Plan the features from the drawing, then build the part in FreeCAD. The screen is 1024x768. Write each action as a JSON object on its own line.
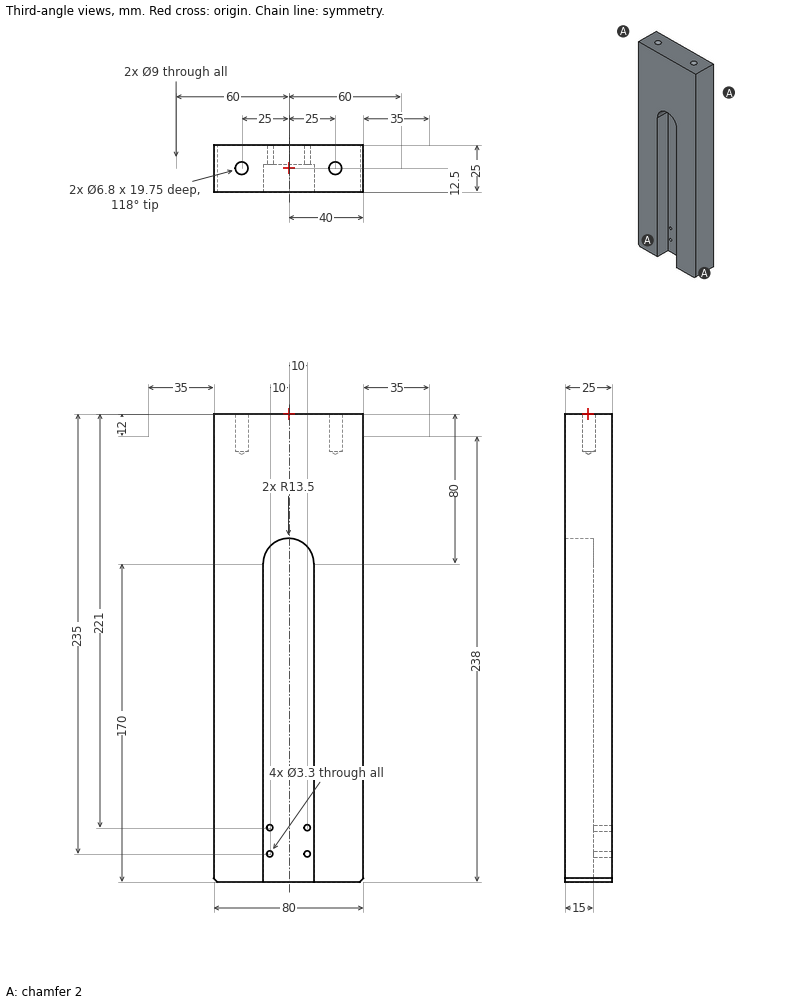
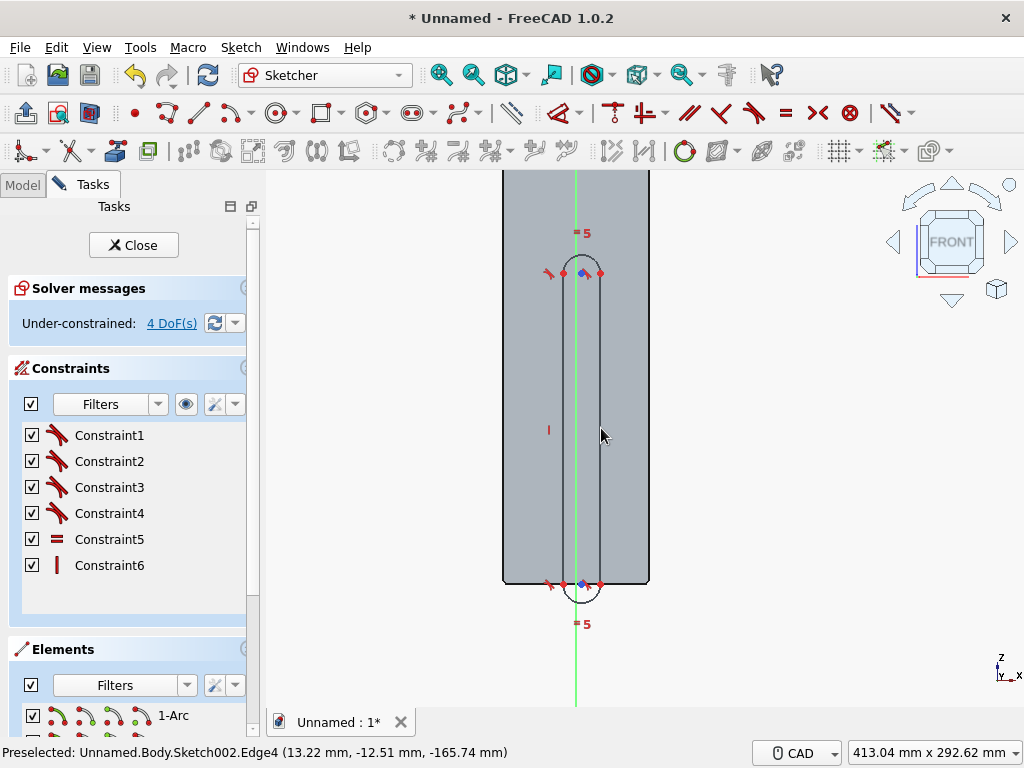
{"action": "left_click", "coordinate": [582, 585]}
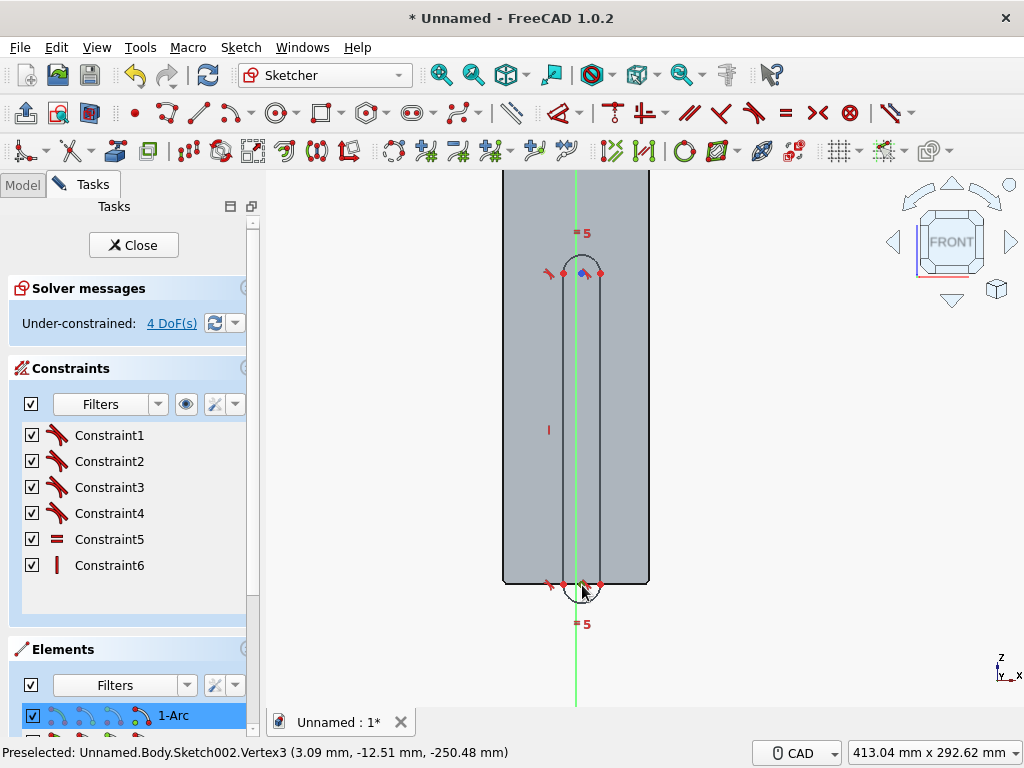
{"action": "left_click", "coordinate": [576, 645]}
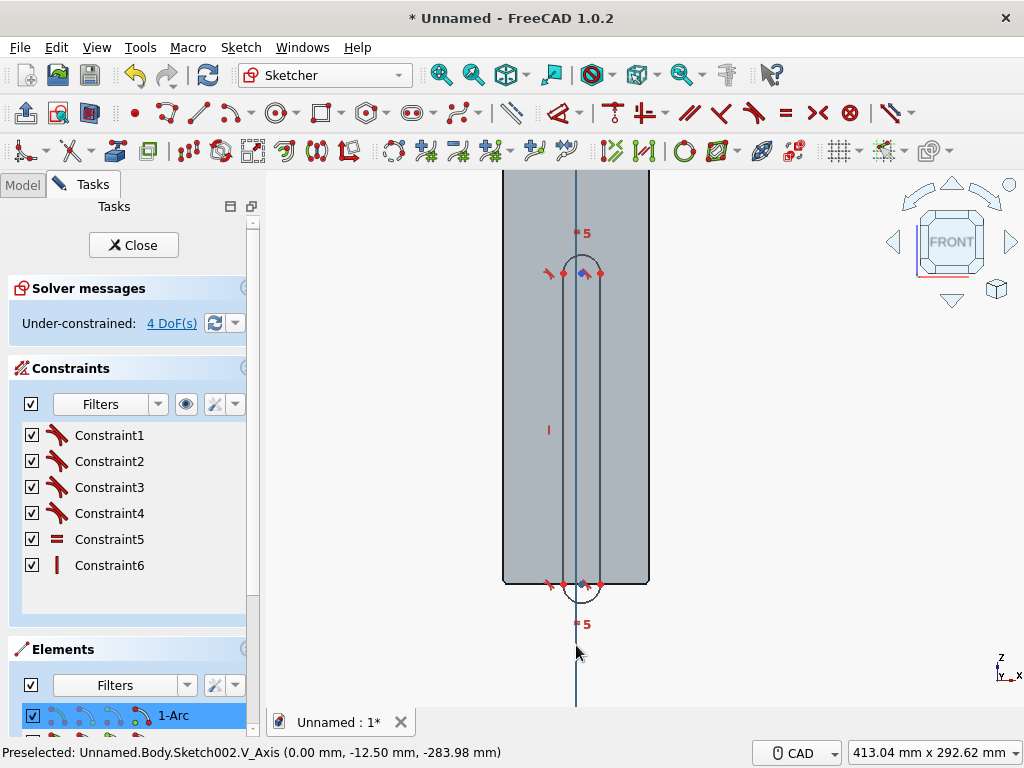
{"action": "left_click", "coordinate": [614, 114]}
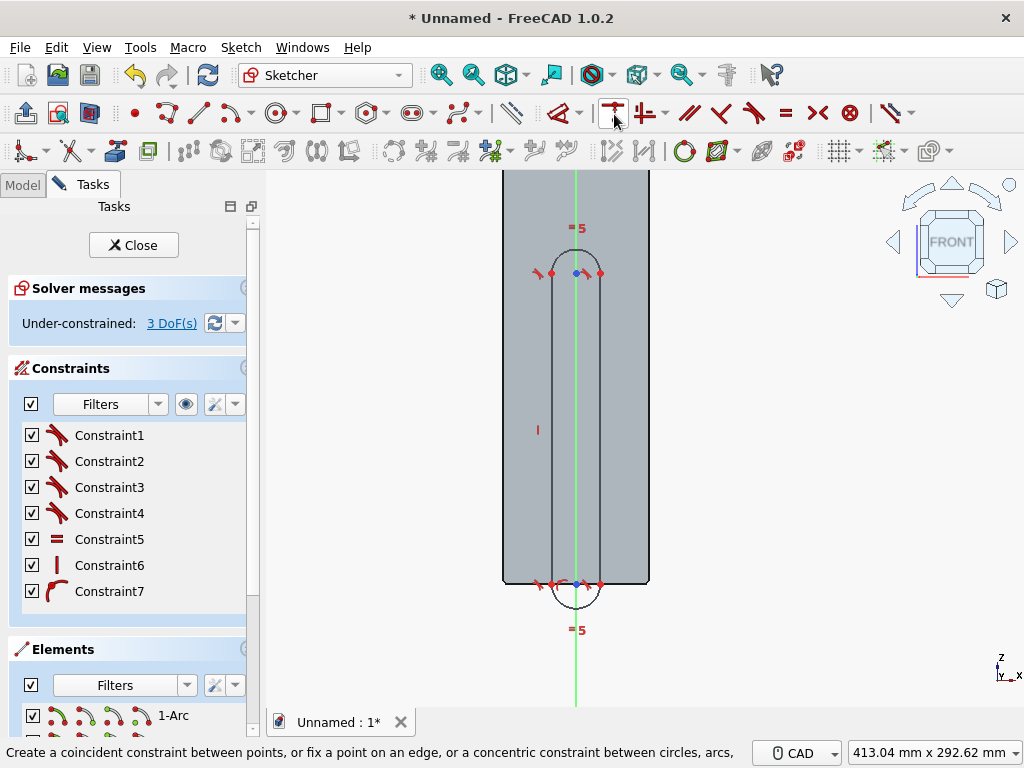
{"action": "left_click", "coordinate": [558, 114]}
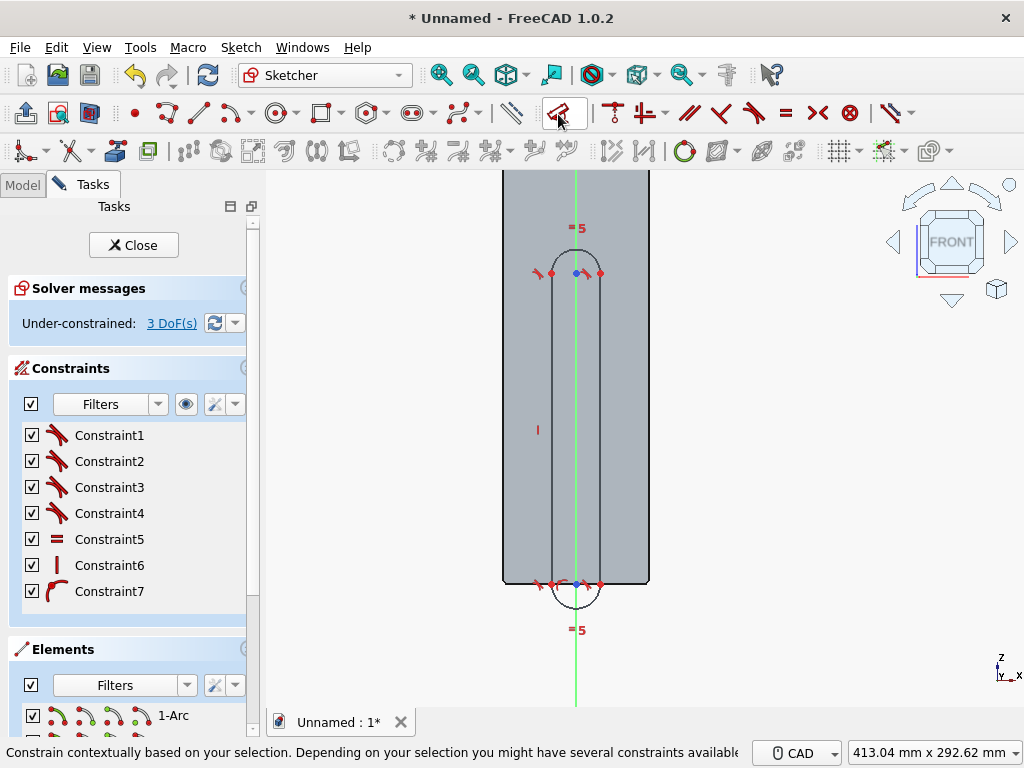
{"action": "scroll", "coordinate": [562, 604], "scroll_direction": "up", "scroll_amount": 3}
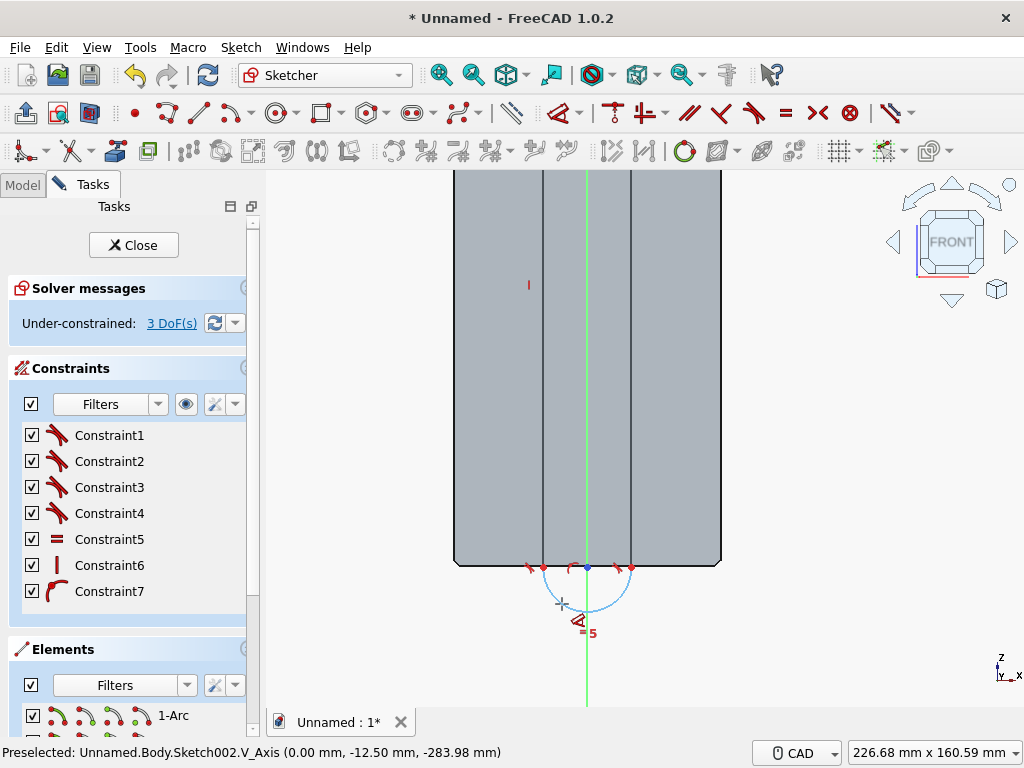
{"action": "left_click", "coordinate": [561, 603]}
{"action": "left_click", "coordinate": [542, 629]}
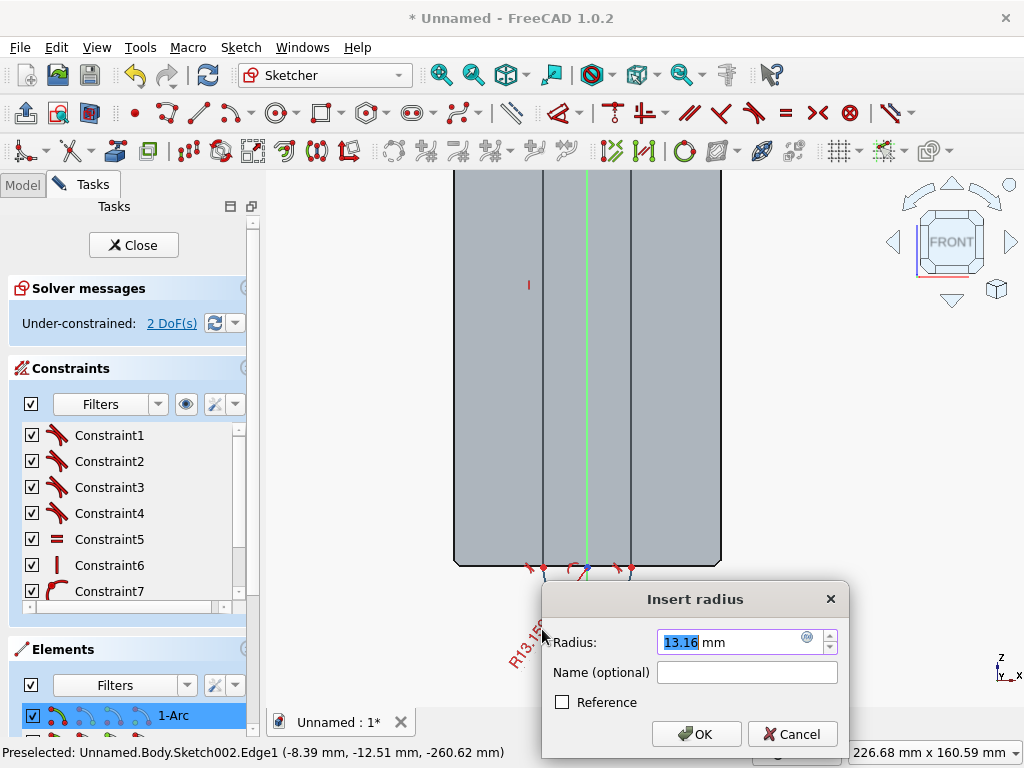
{"action": "type", "text": "13.5"}
{"action": "key", "text": "Return"}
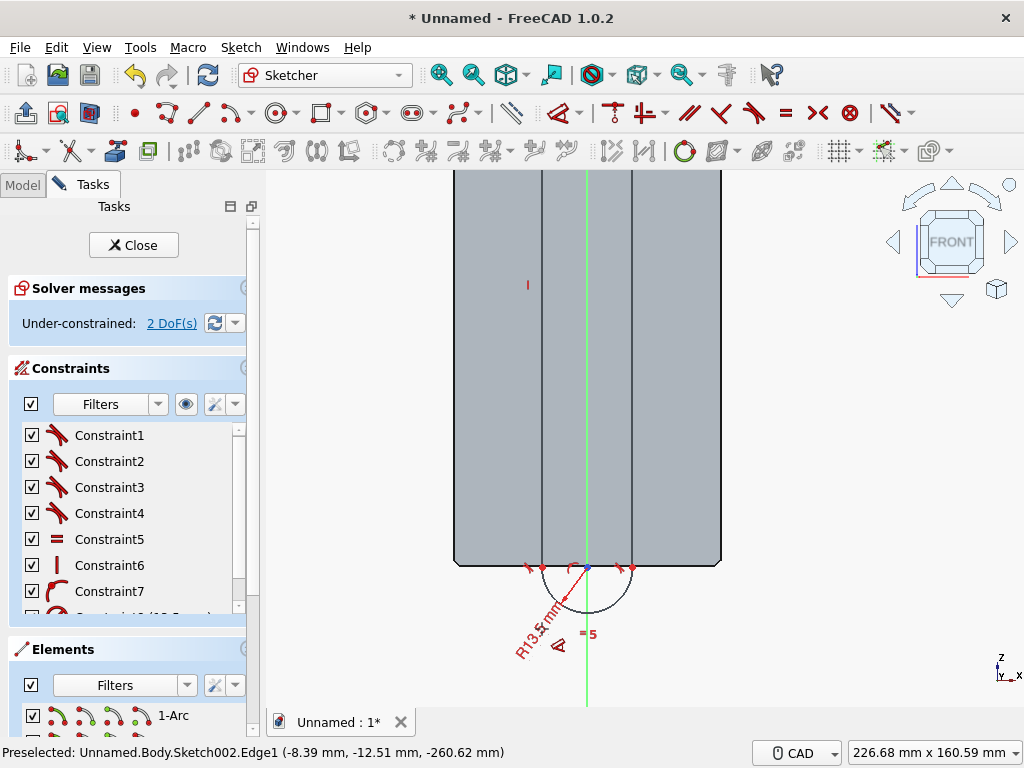
{"action": "left_click", "coordinate": [542, 398]}
{"action": "left_click", "coordinate": [508, 383]}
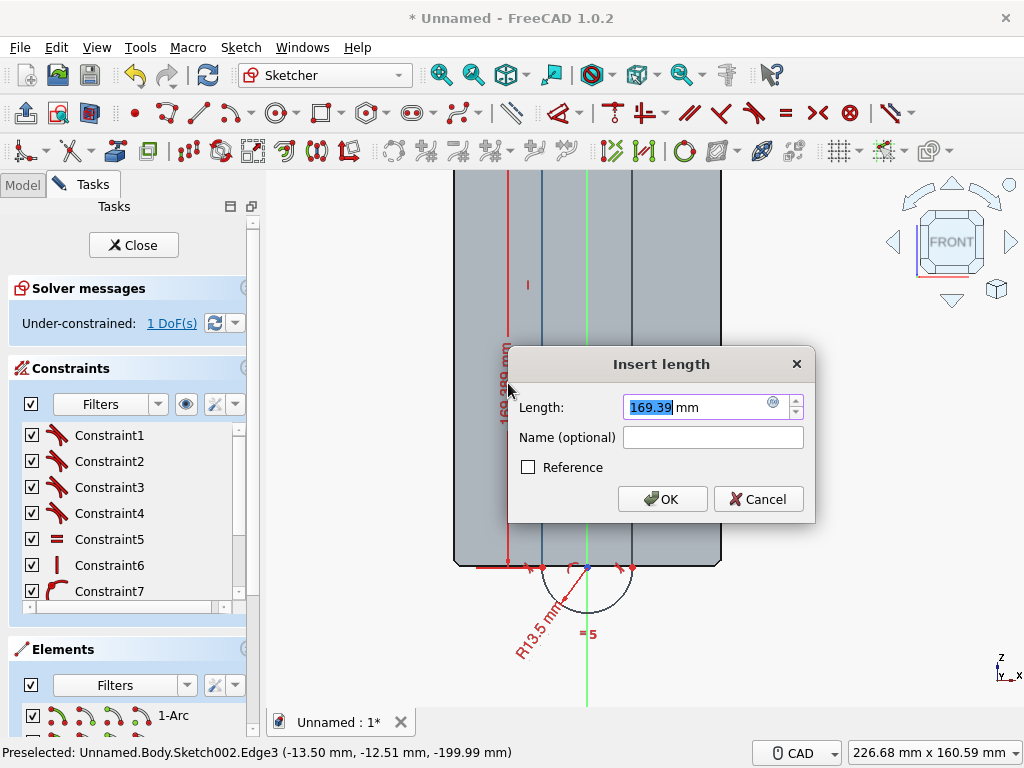
{"action": "type", "text": "170"}
{"action": "key", "text": "Return"}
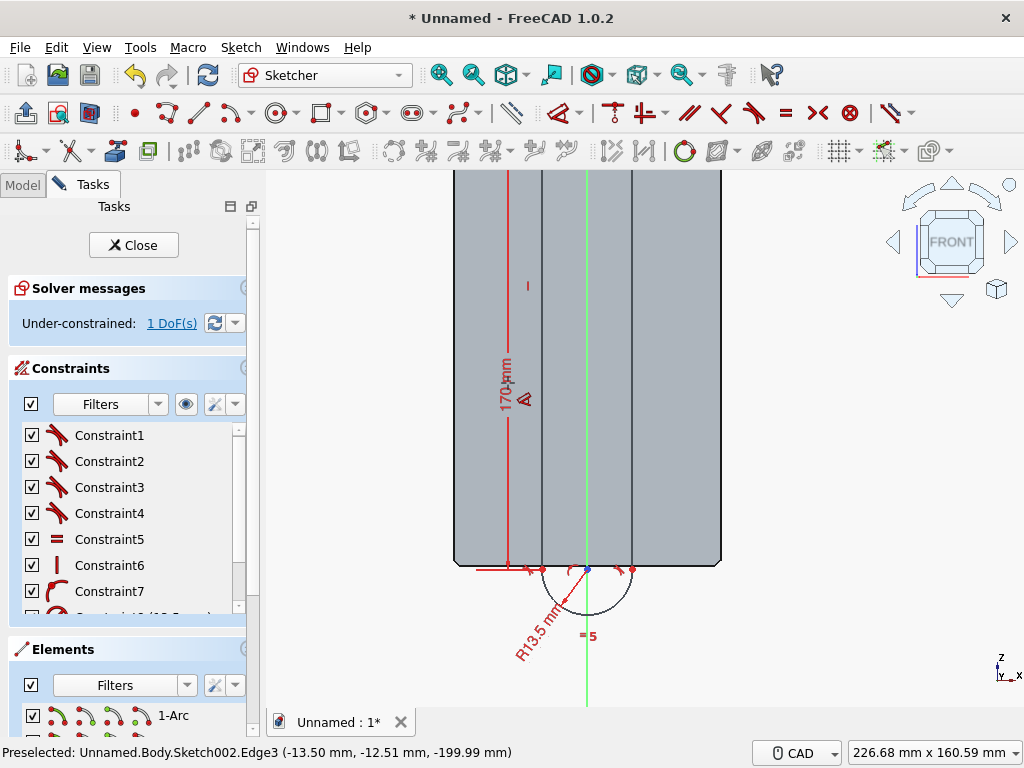
{"action": "scroll", "coordinate": [570, 594], "scroll_direction": "down", "scroll_amount": 5}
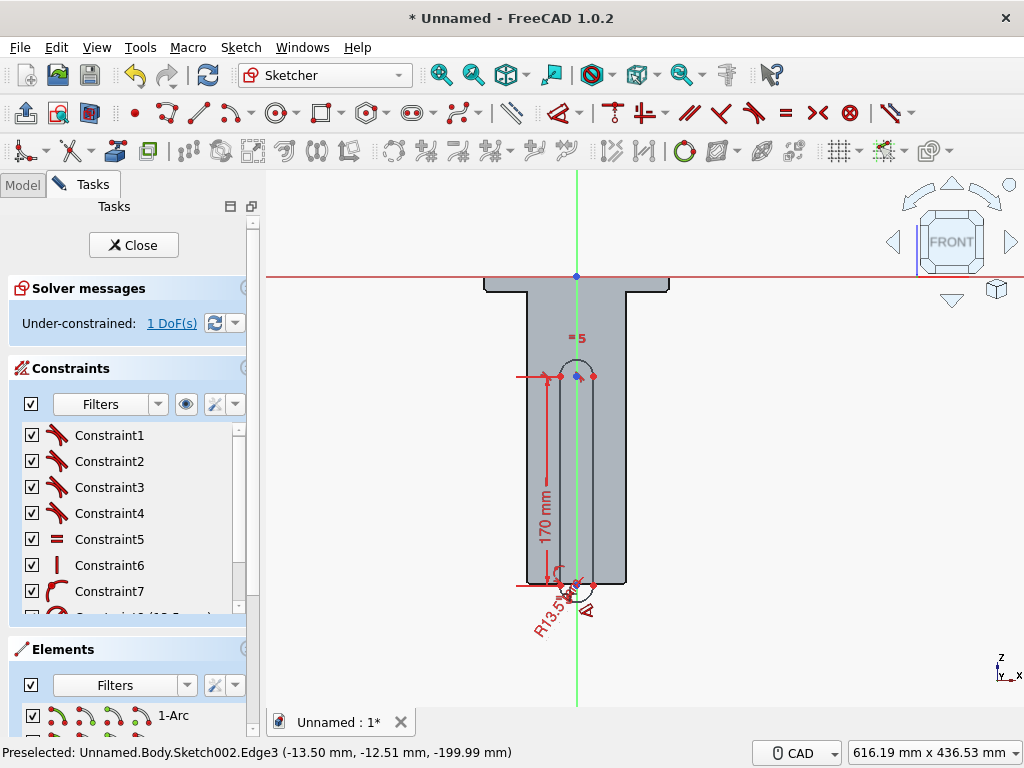
{"action": "left_click", "coordinate": [593, 377]}
{"action": "left_click", "coordinate": [627, 327]}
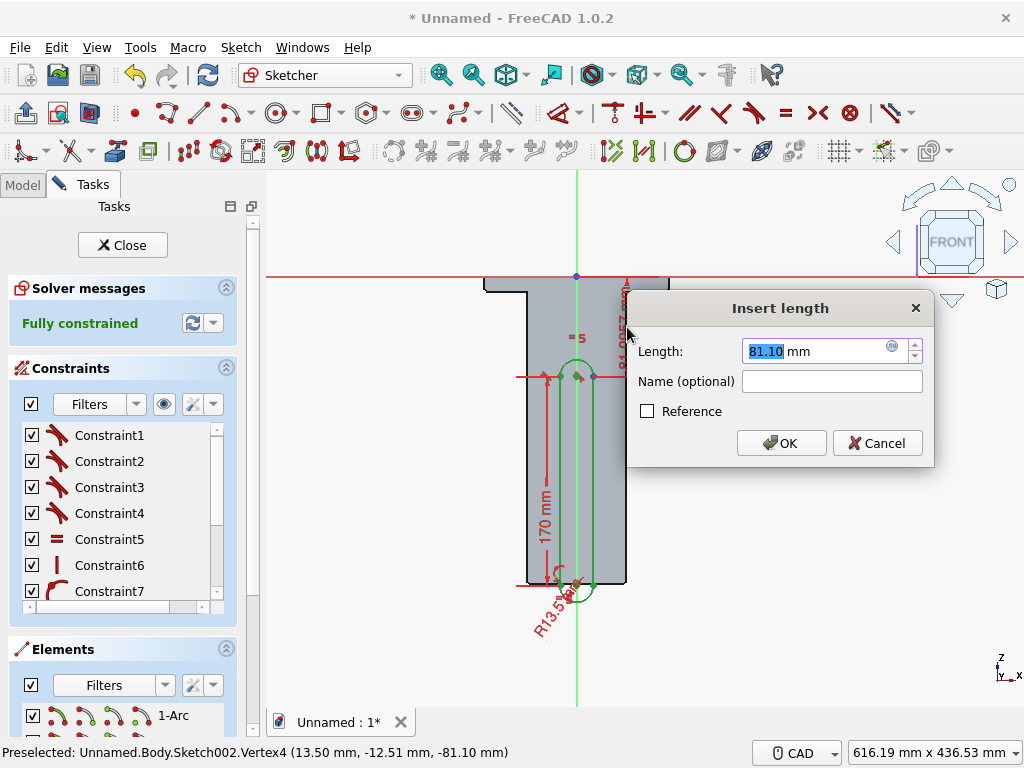
{"action": "type", "text": "80"}
{"action": "key", "text": "Return"}
{"action": "key", "text": "Escape"}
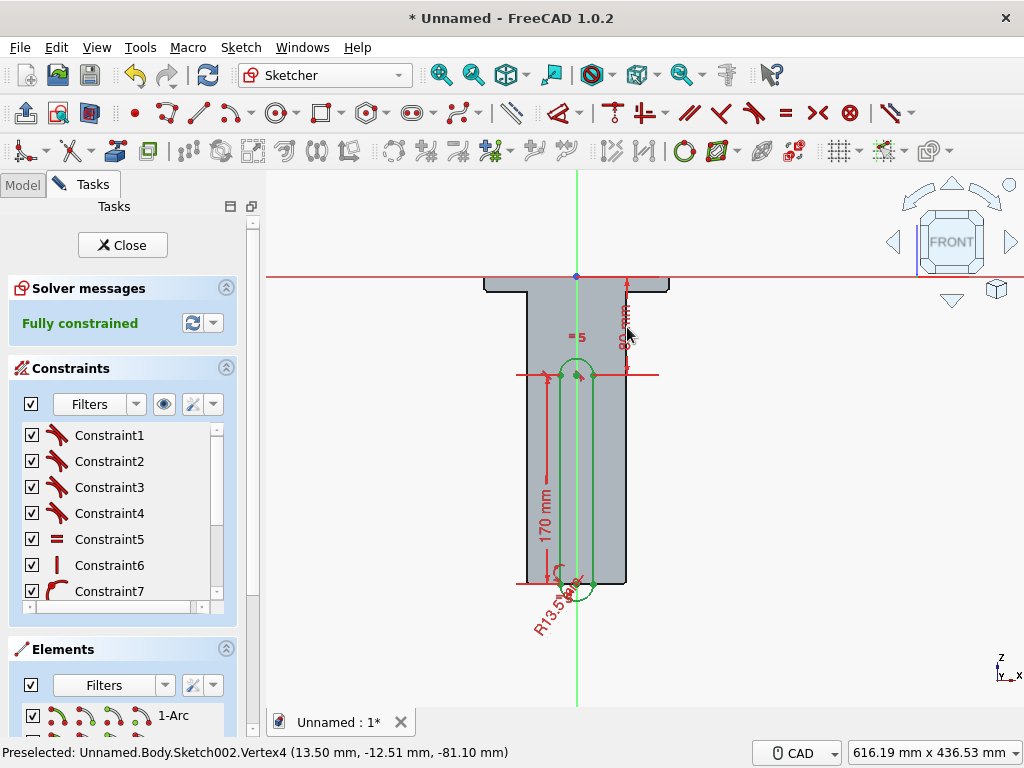
{"action": "left_click", "coordinate": [123, 245]}